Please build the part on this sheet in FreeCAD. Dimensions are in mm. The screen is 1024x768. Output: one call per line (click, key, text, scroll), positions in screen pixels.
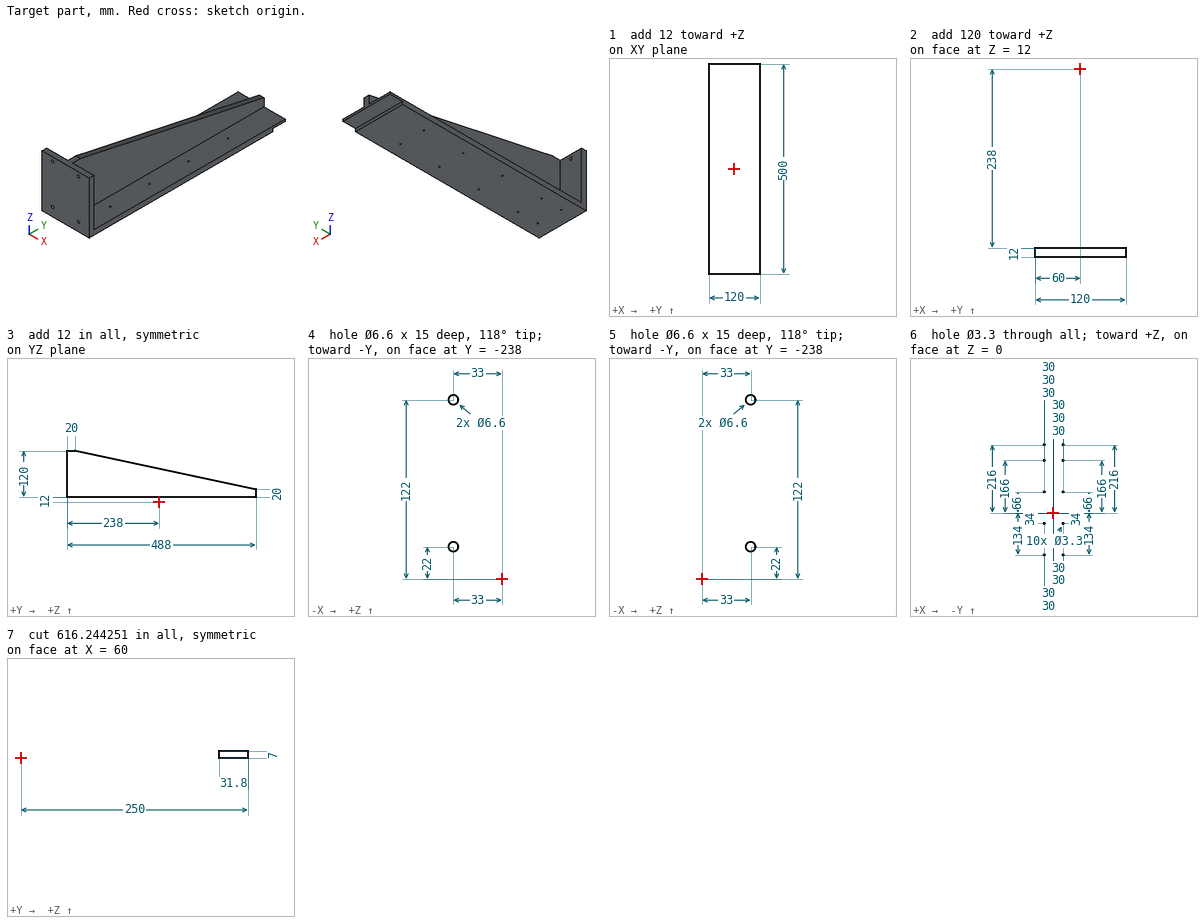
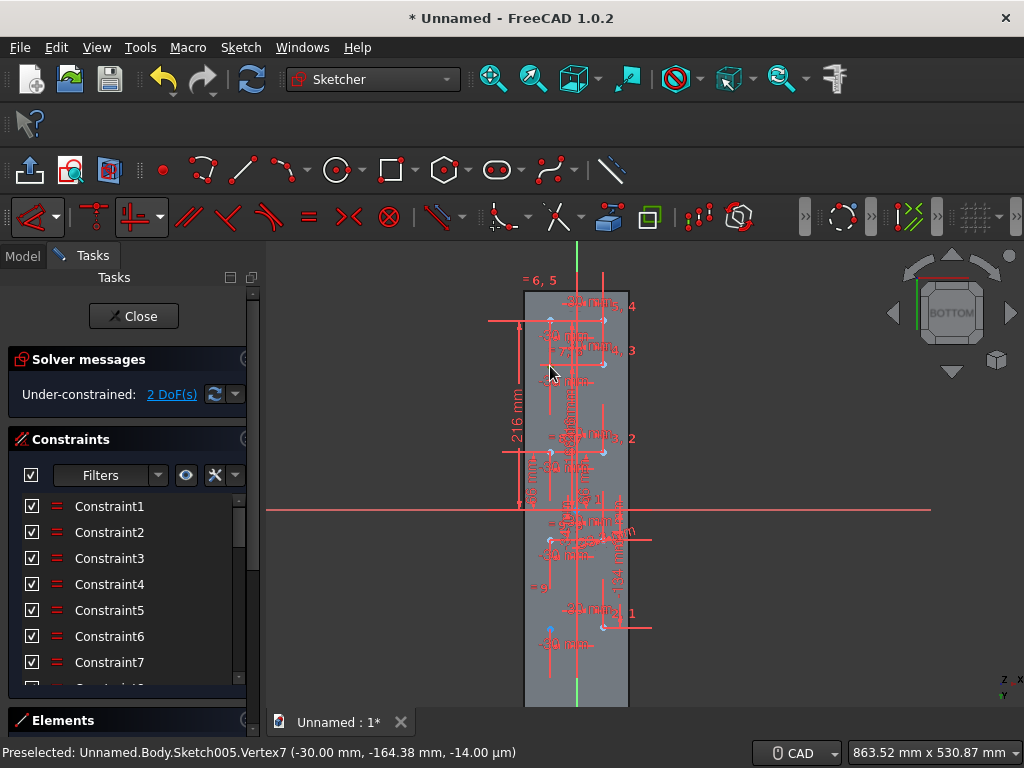
click(58, 218)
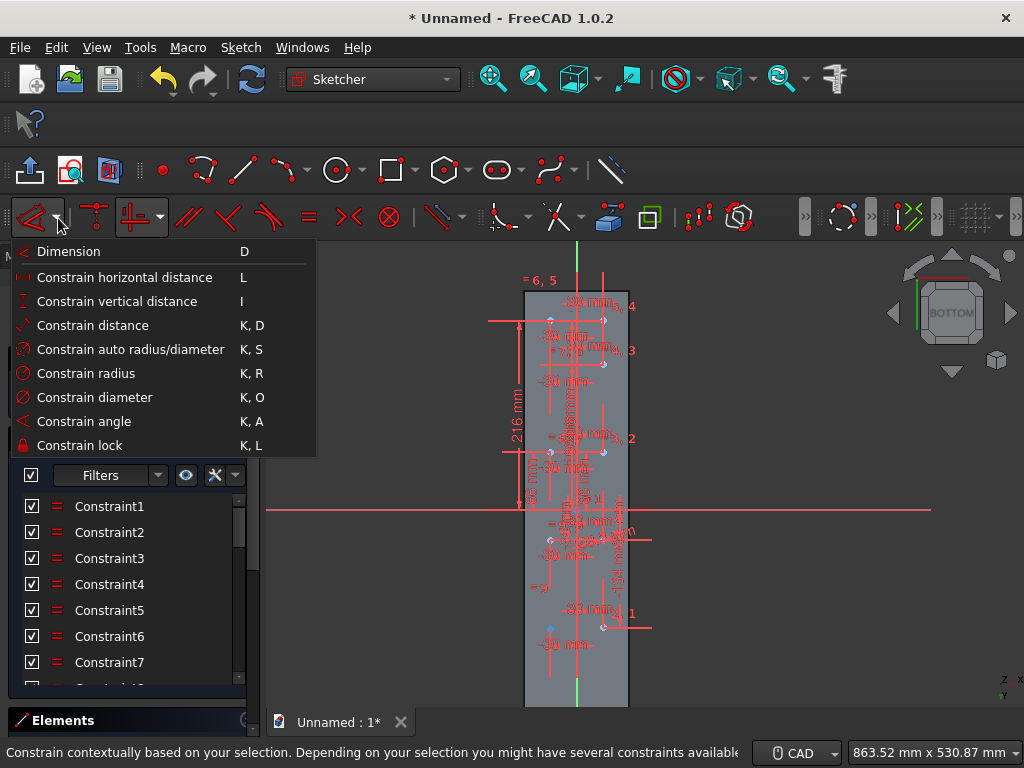
click(164, 301)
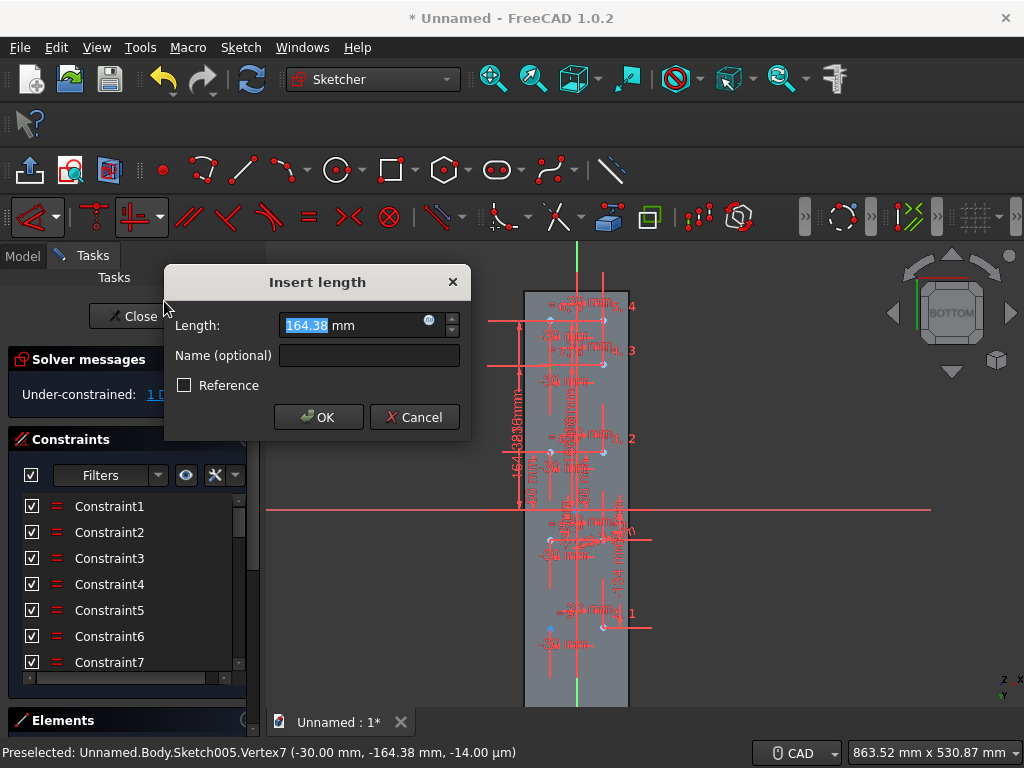
text(166)
key(Return)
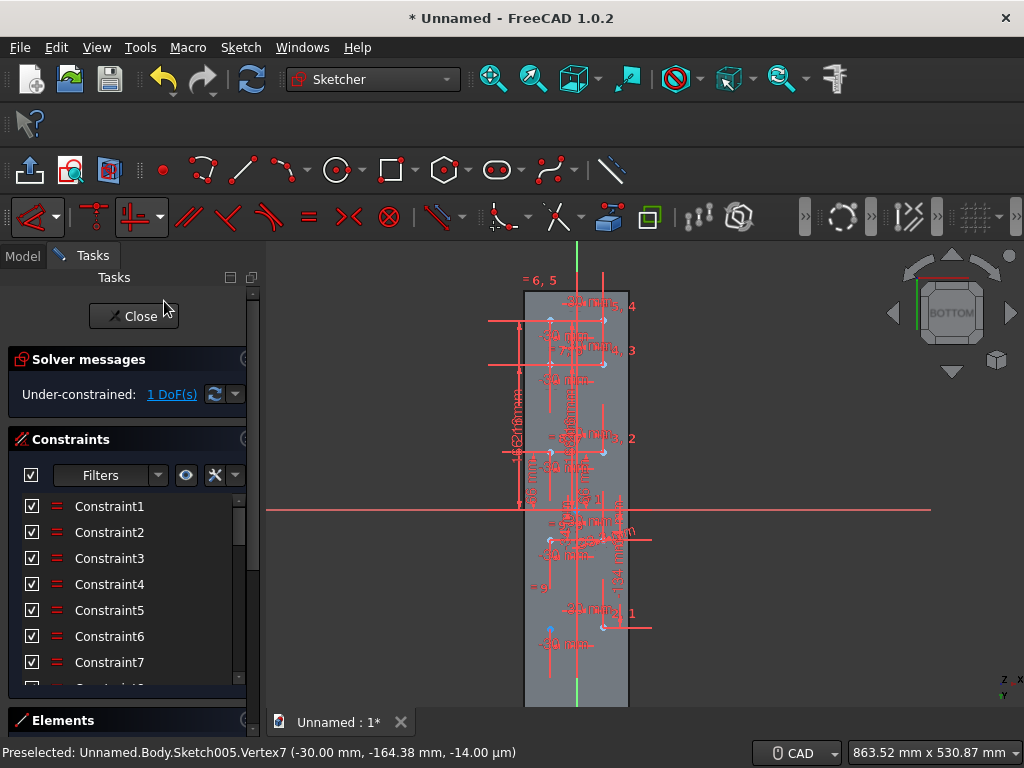
click(550, 629)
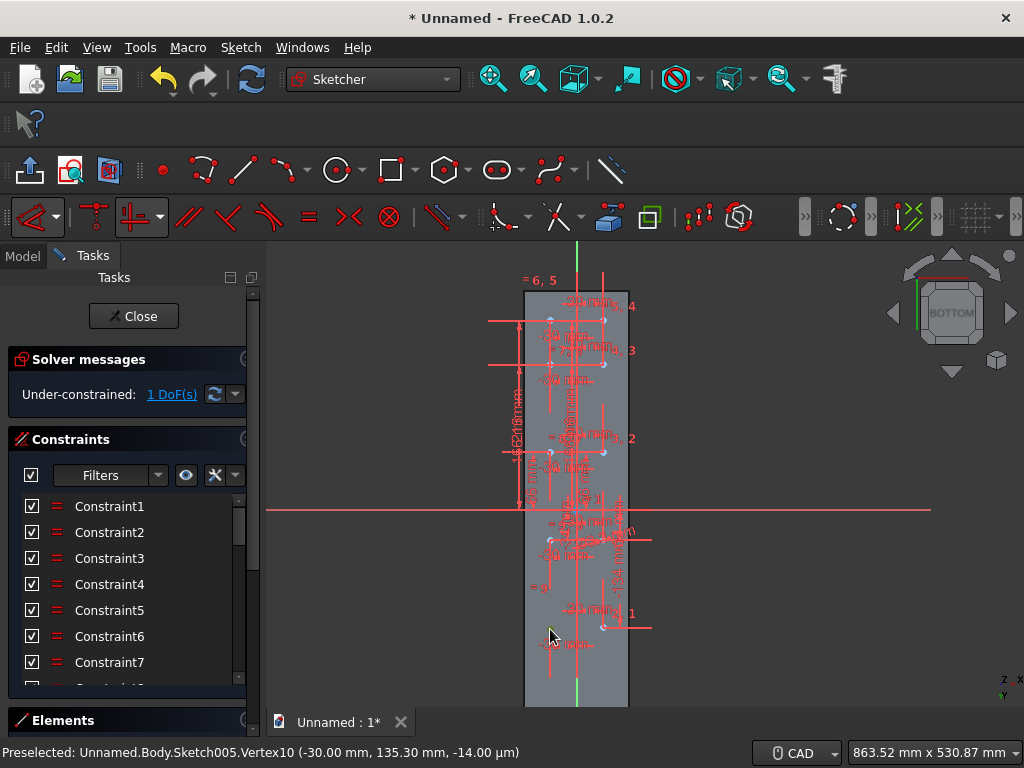
key(i)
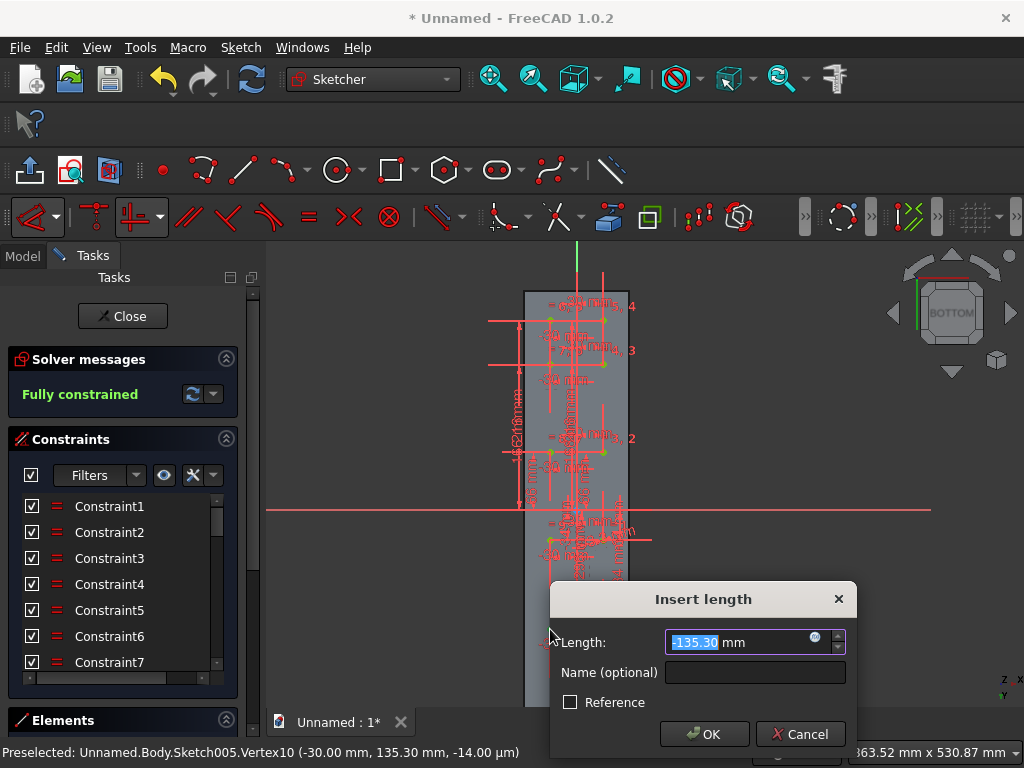
text(-134)
key(Return)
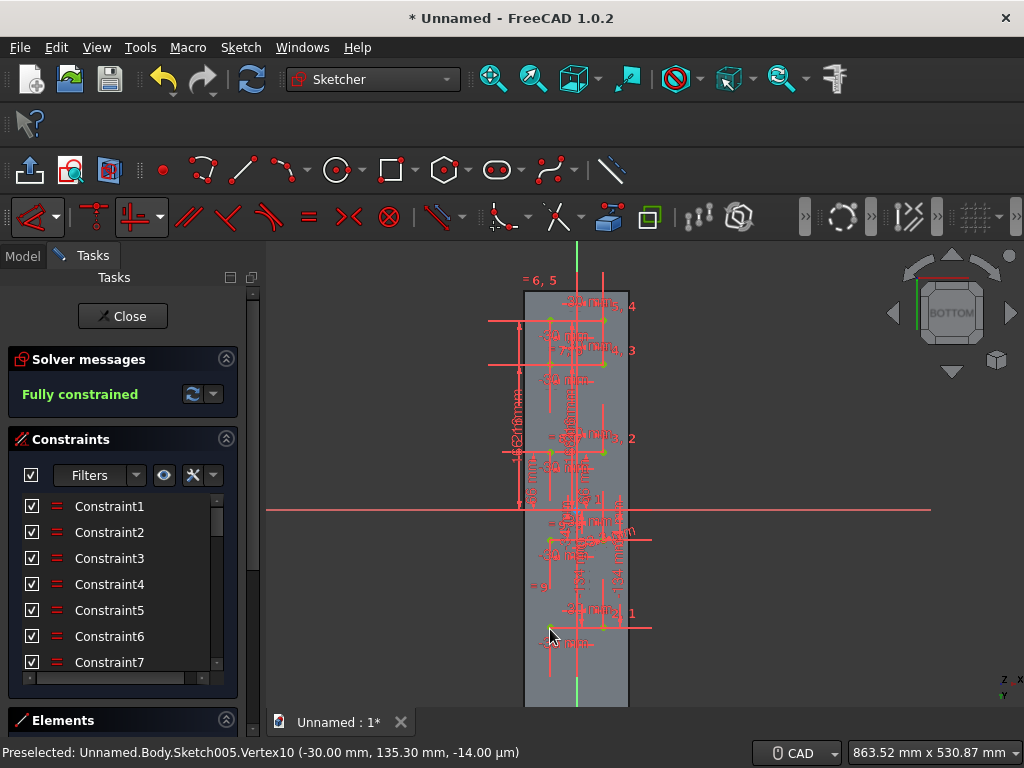
click(123, 316)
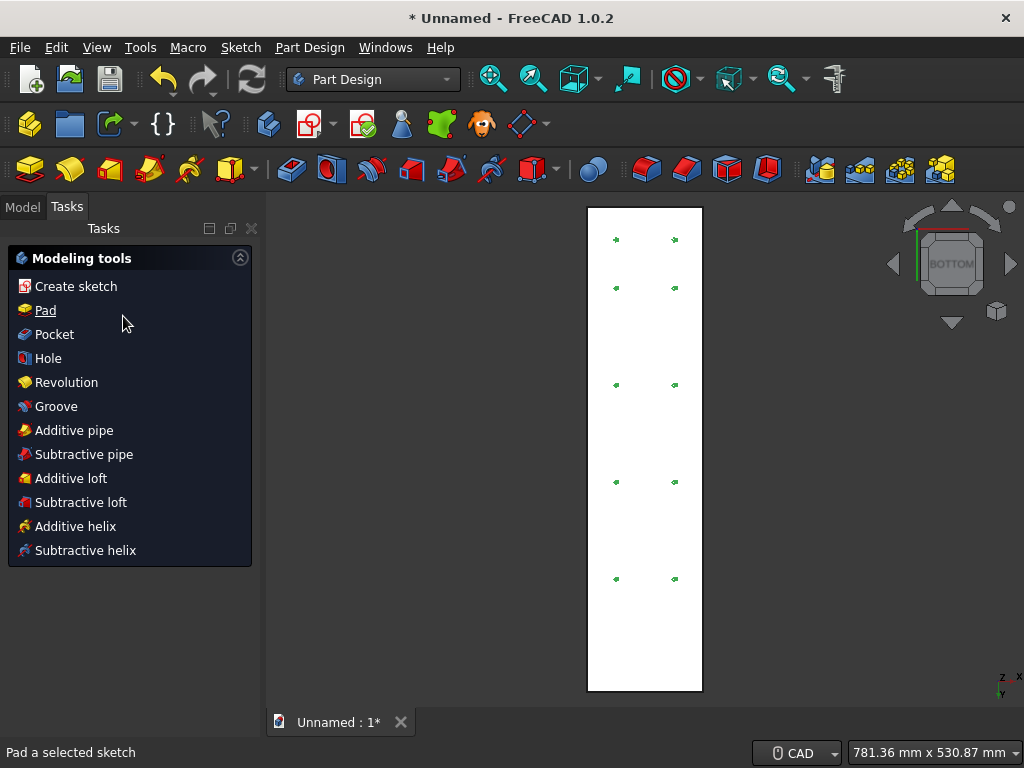
click(332, 170)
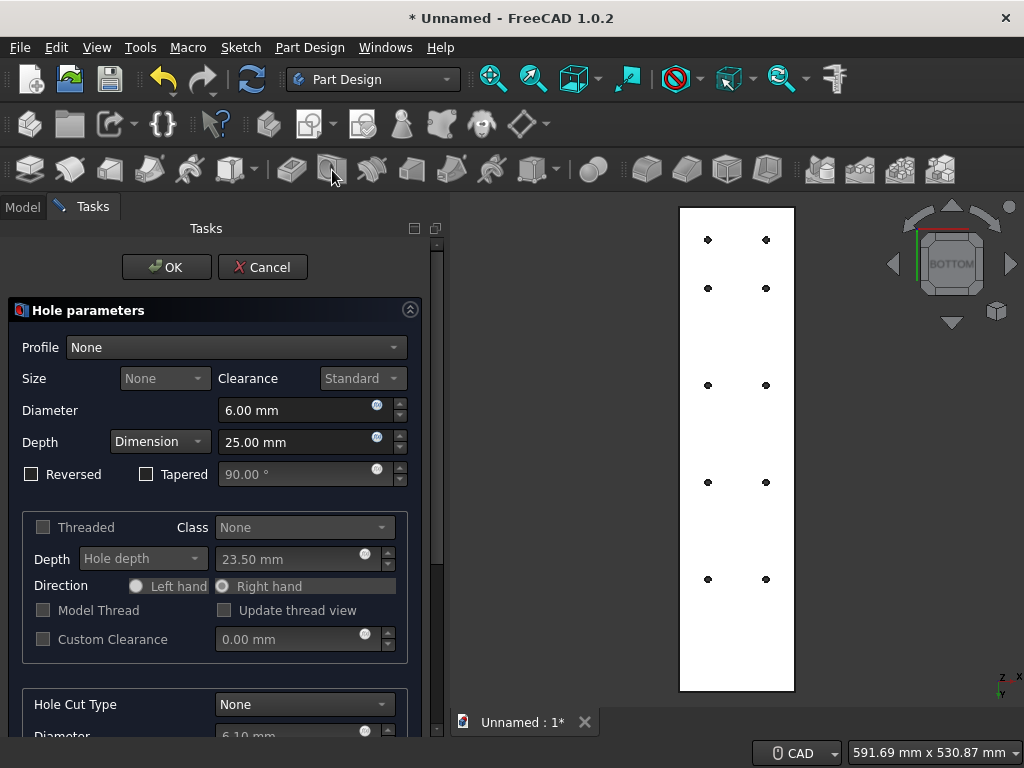
triple_click(305, 410)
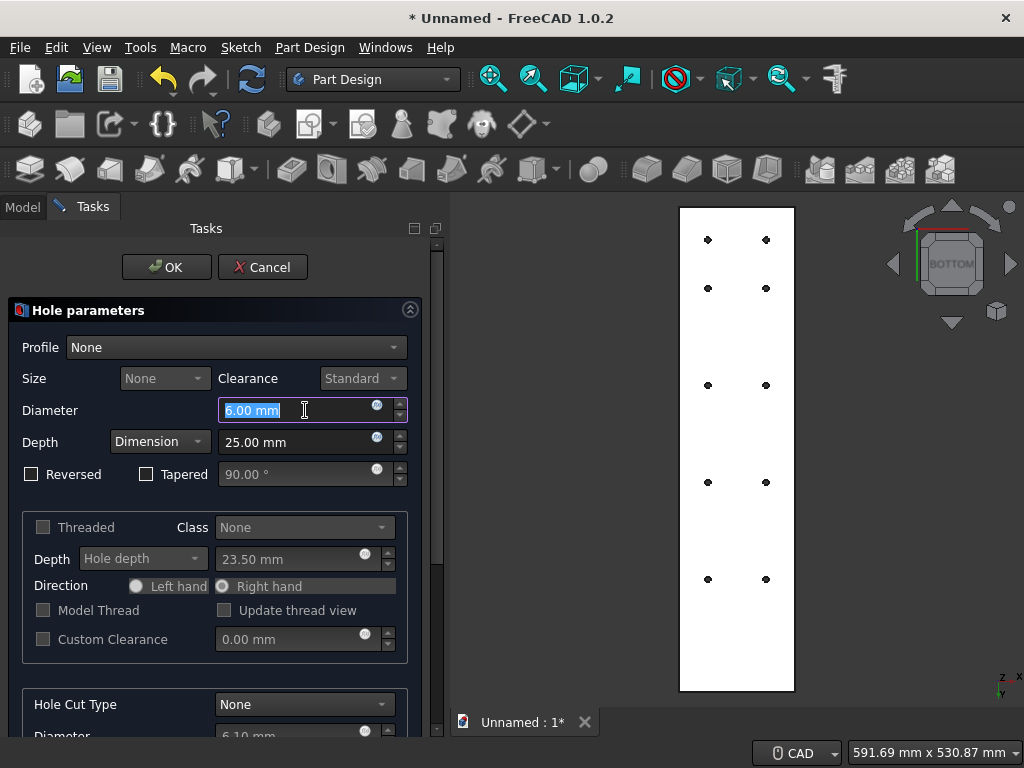
text(3.3)
key(Tab)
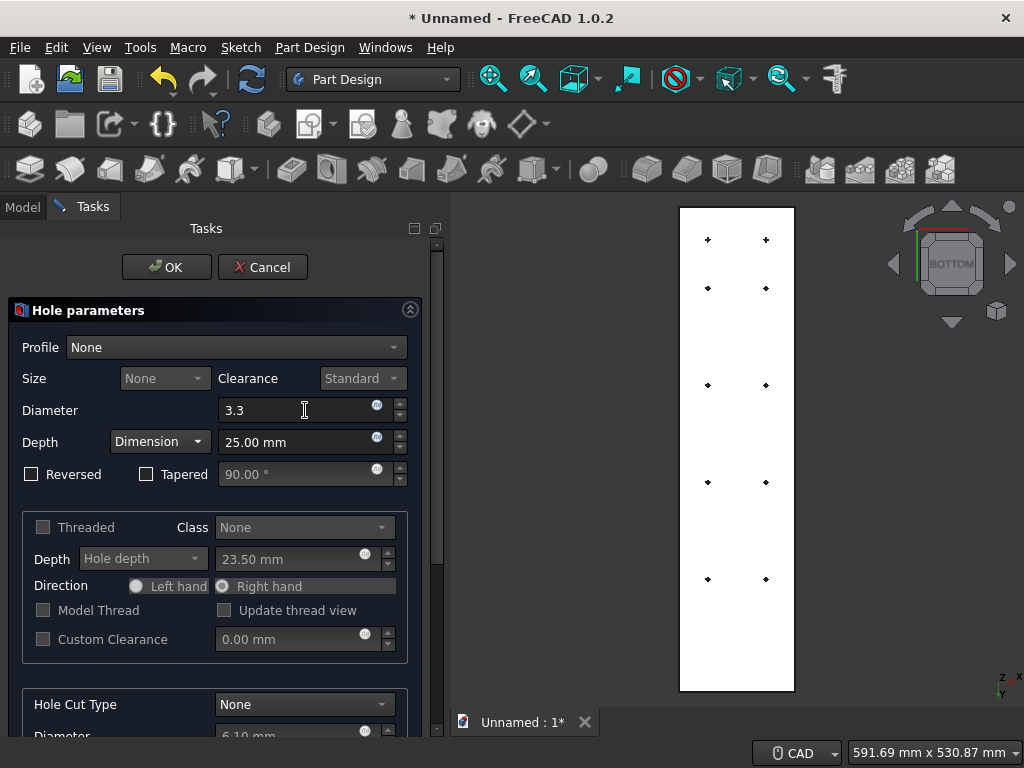
click(161, 442)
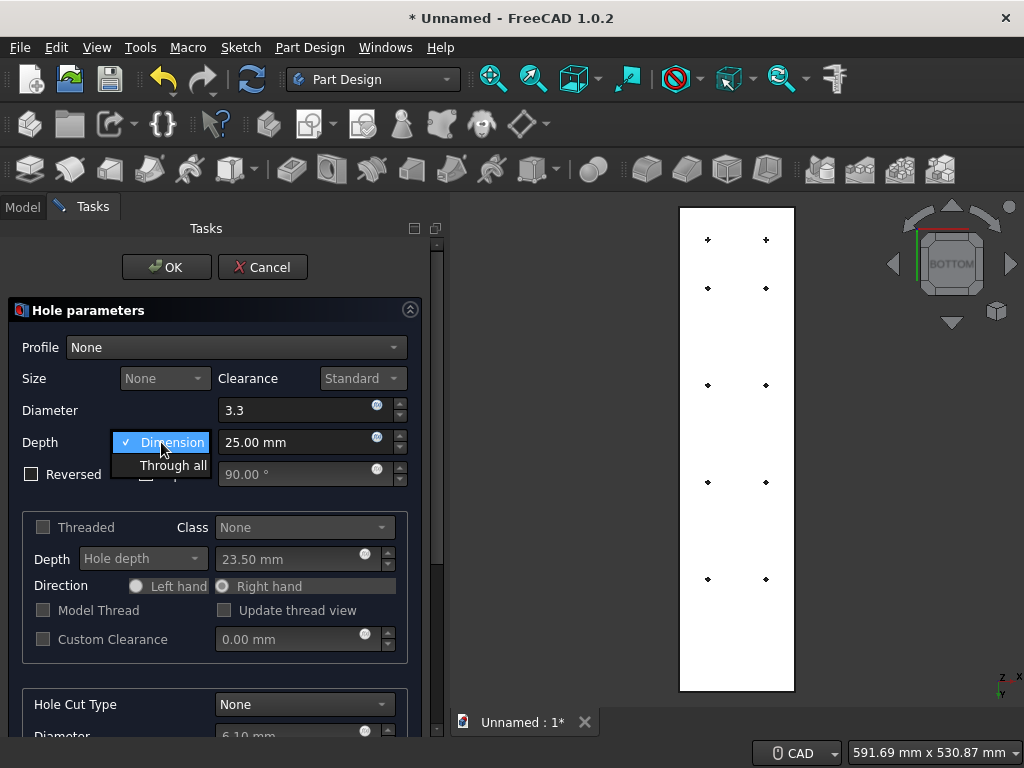
click(160, 466)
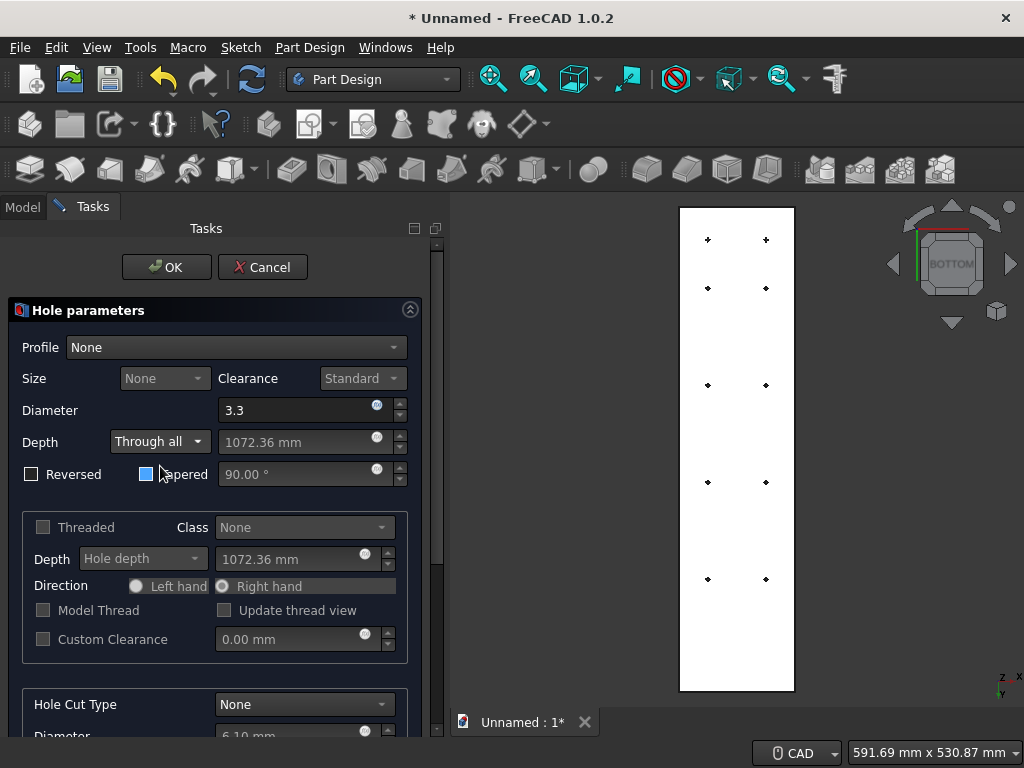
click(167, 267)